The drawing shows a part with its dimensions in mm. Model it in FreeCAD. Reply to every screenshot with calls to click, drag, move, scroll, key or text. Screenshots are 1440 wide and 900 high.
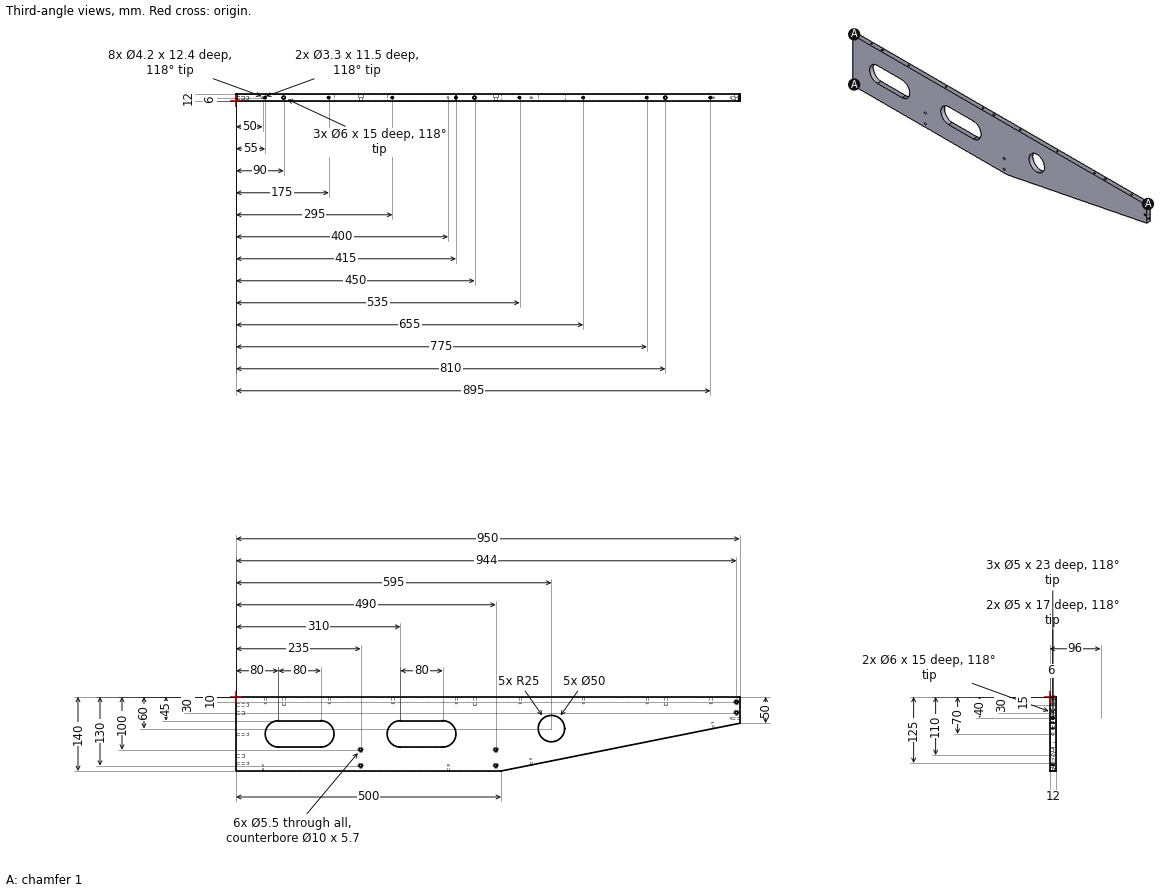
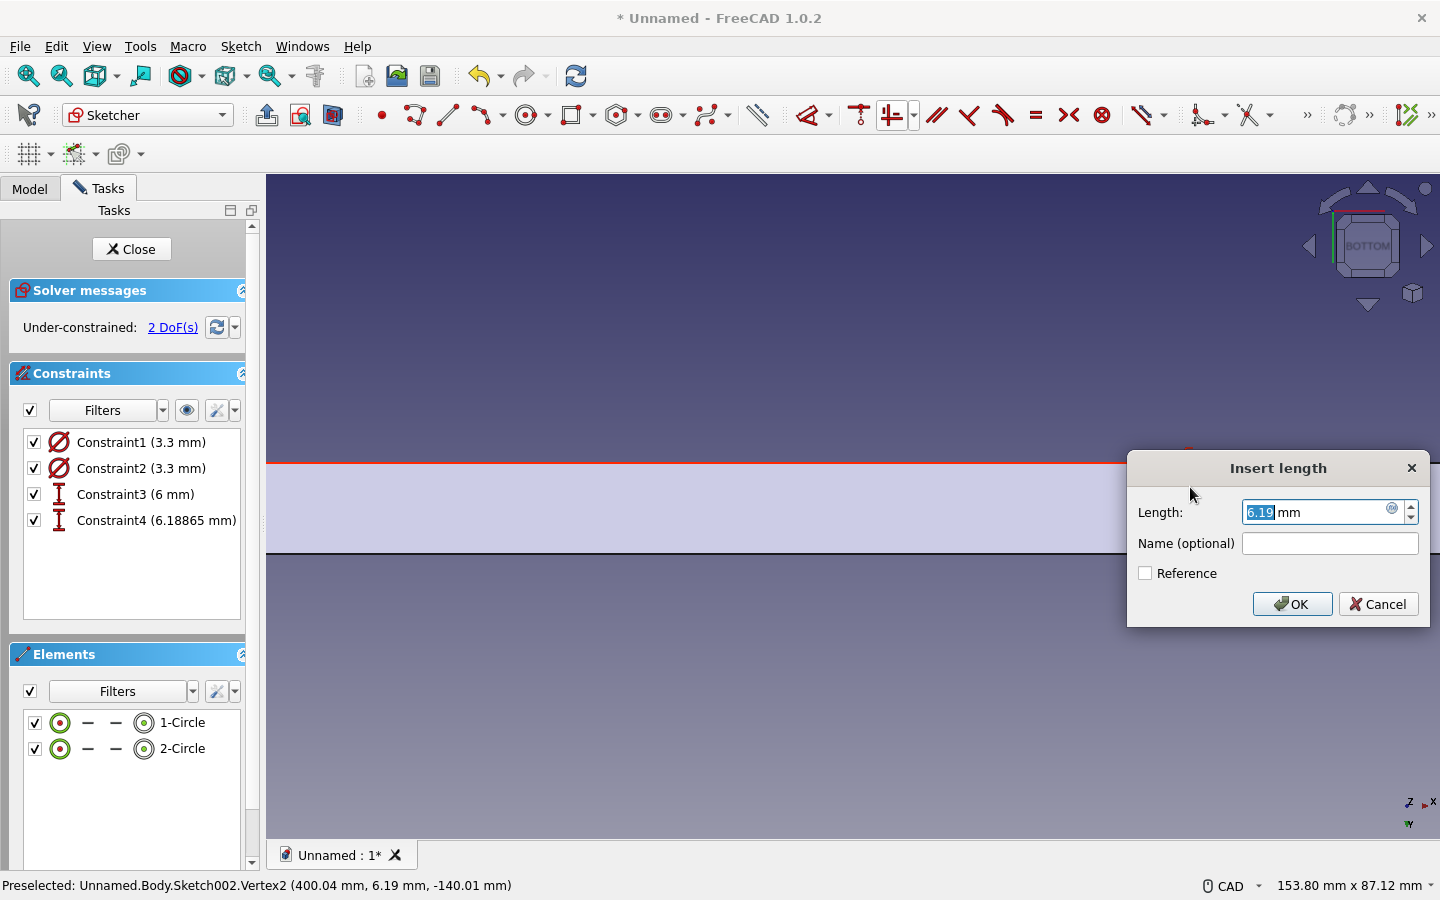
text(6)
key(Return)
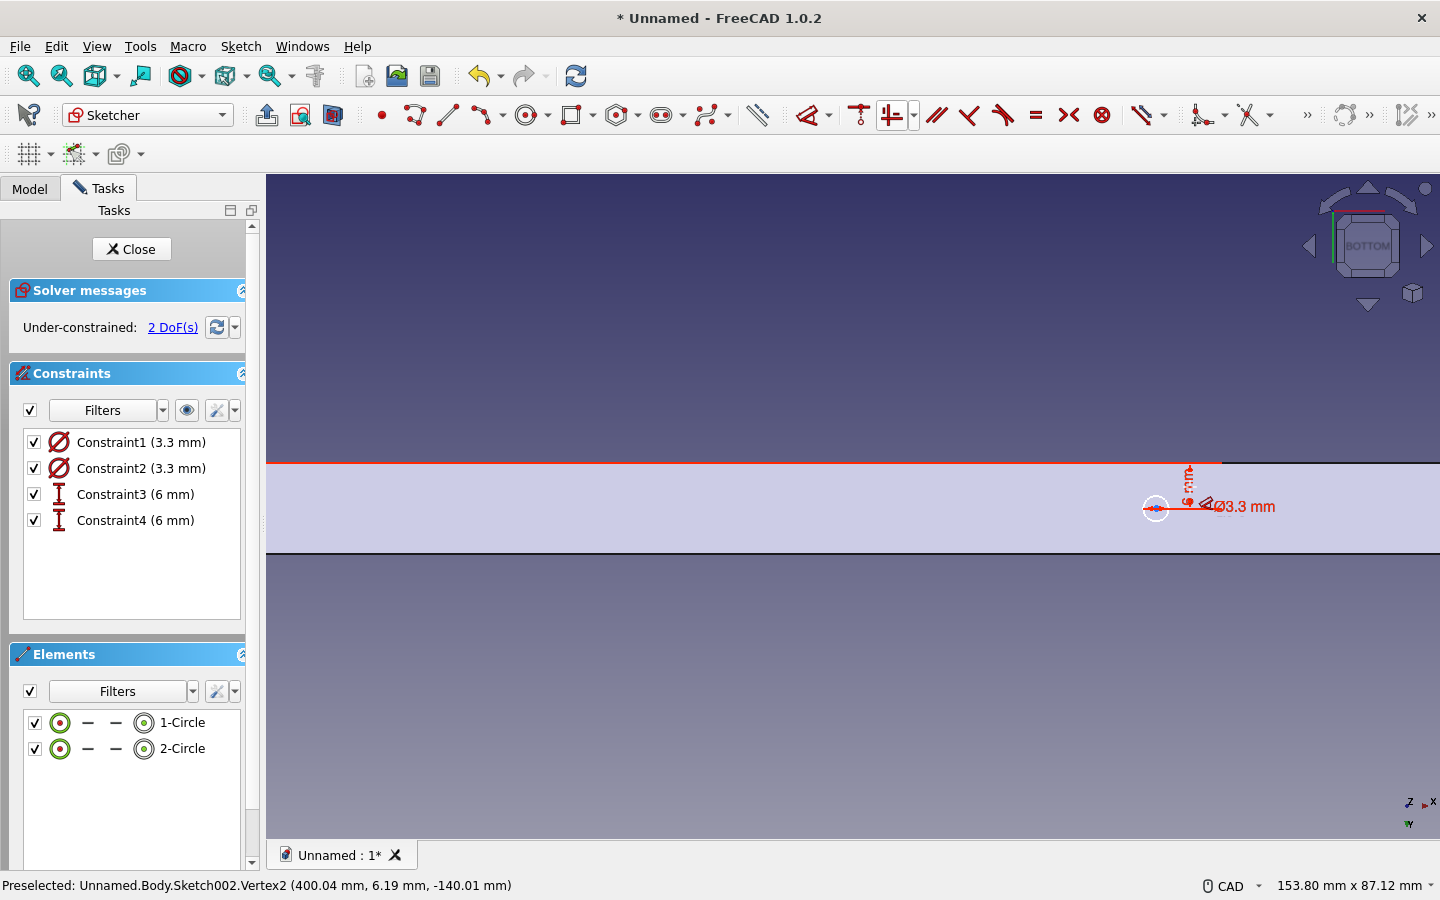
scroll(1161, 511, down, 7)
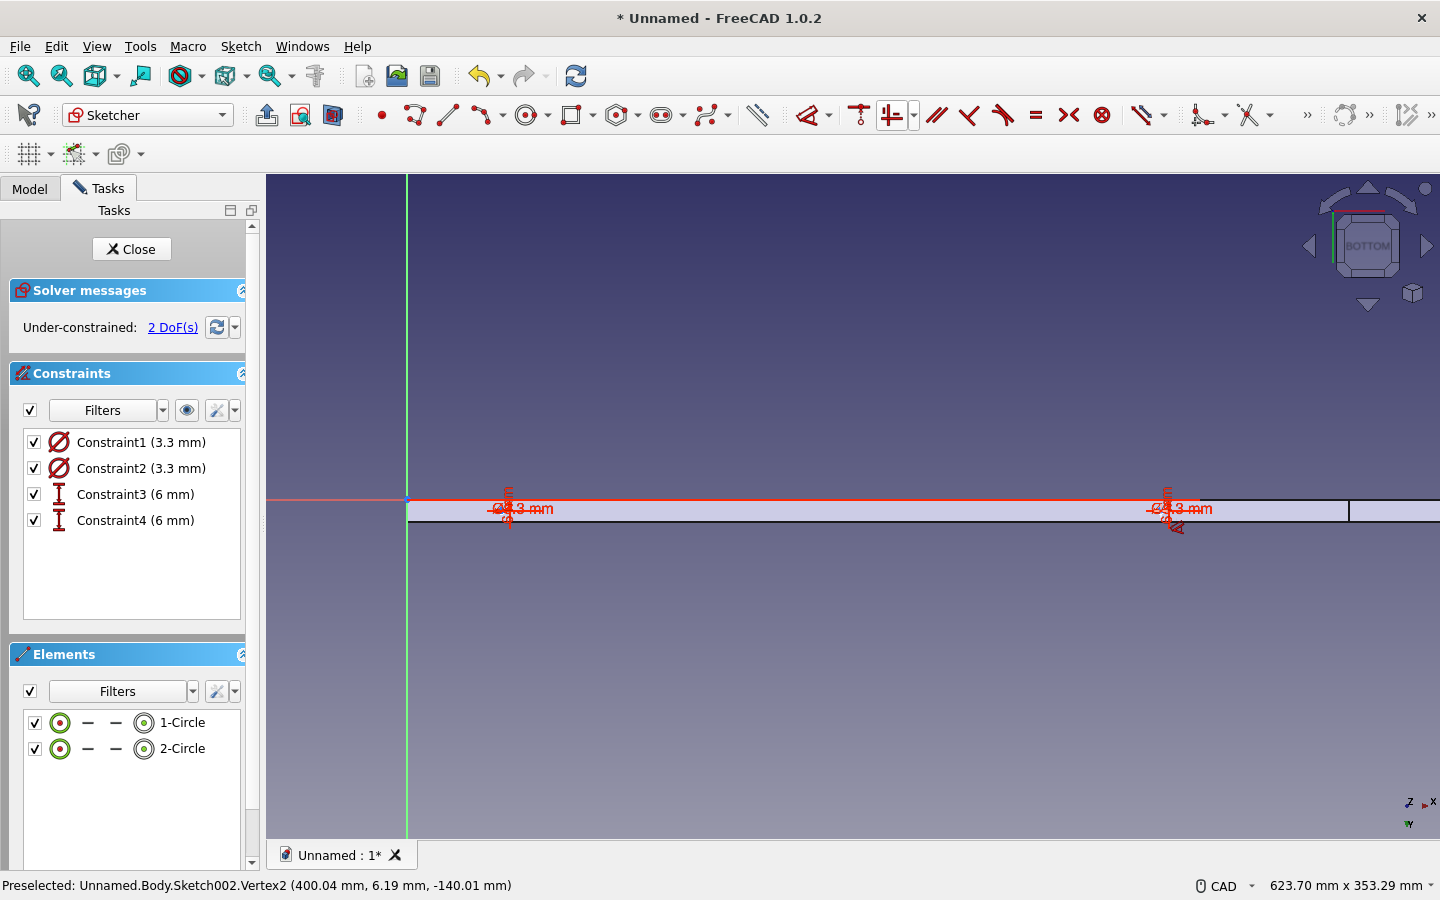
click(501, 511)
click(454, 466)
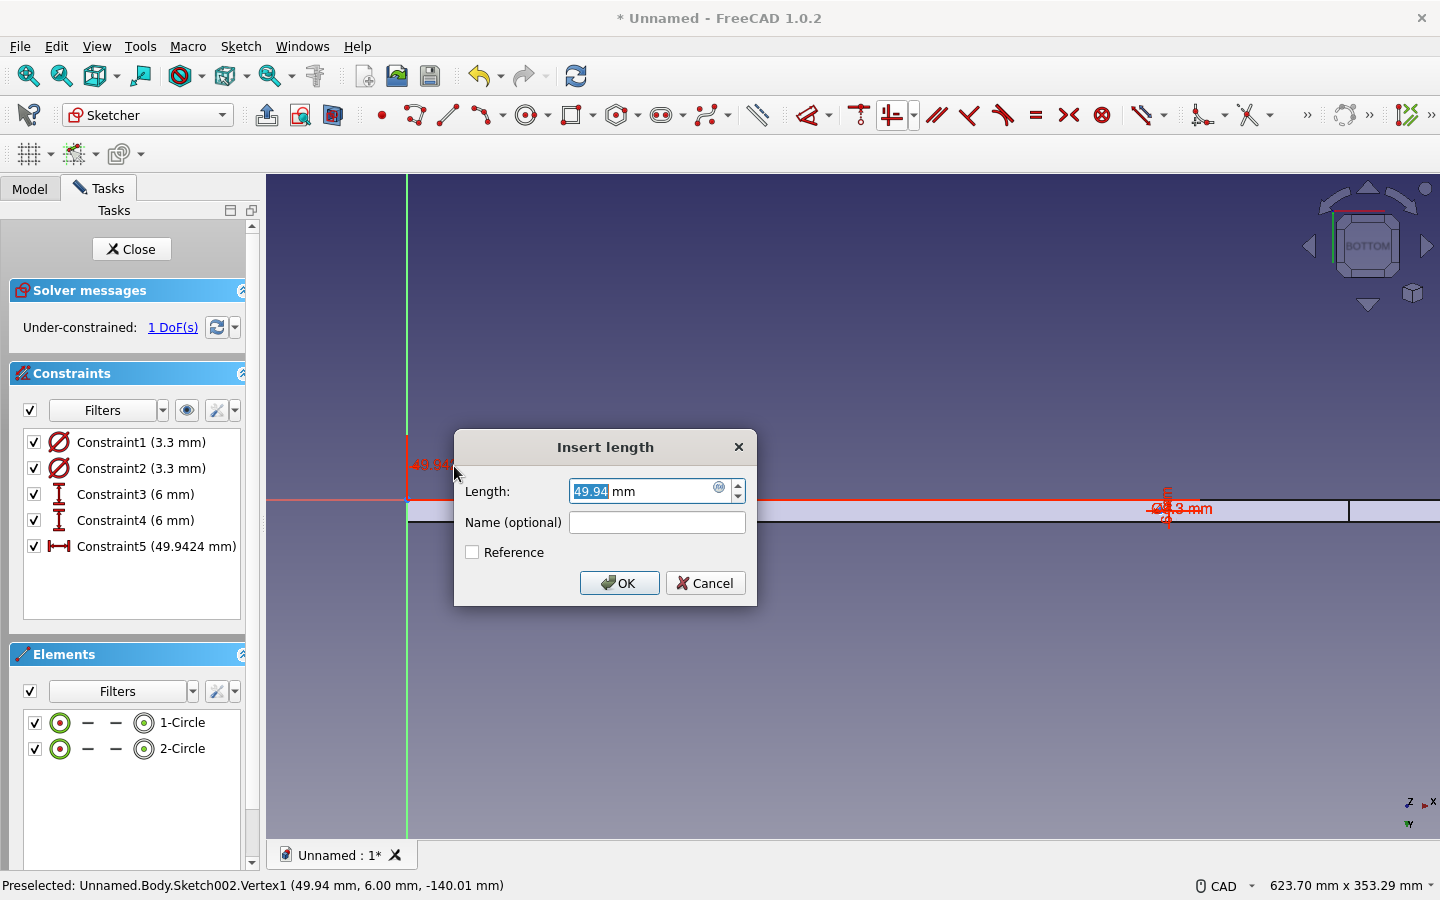
text(50)
key(Return)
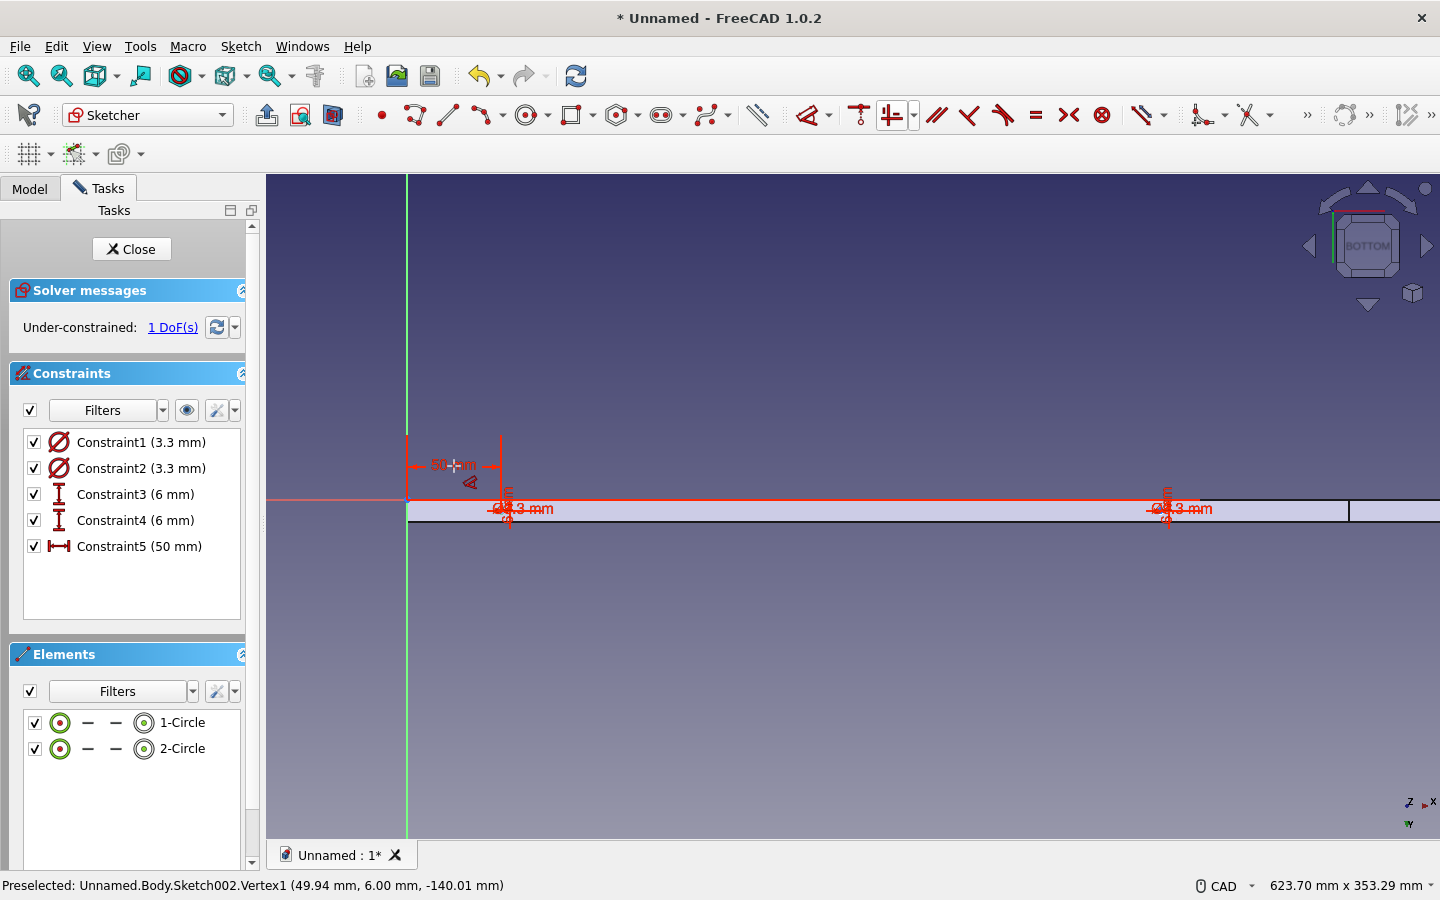
click(1160, 511)
click(784, 466)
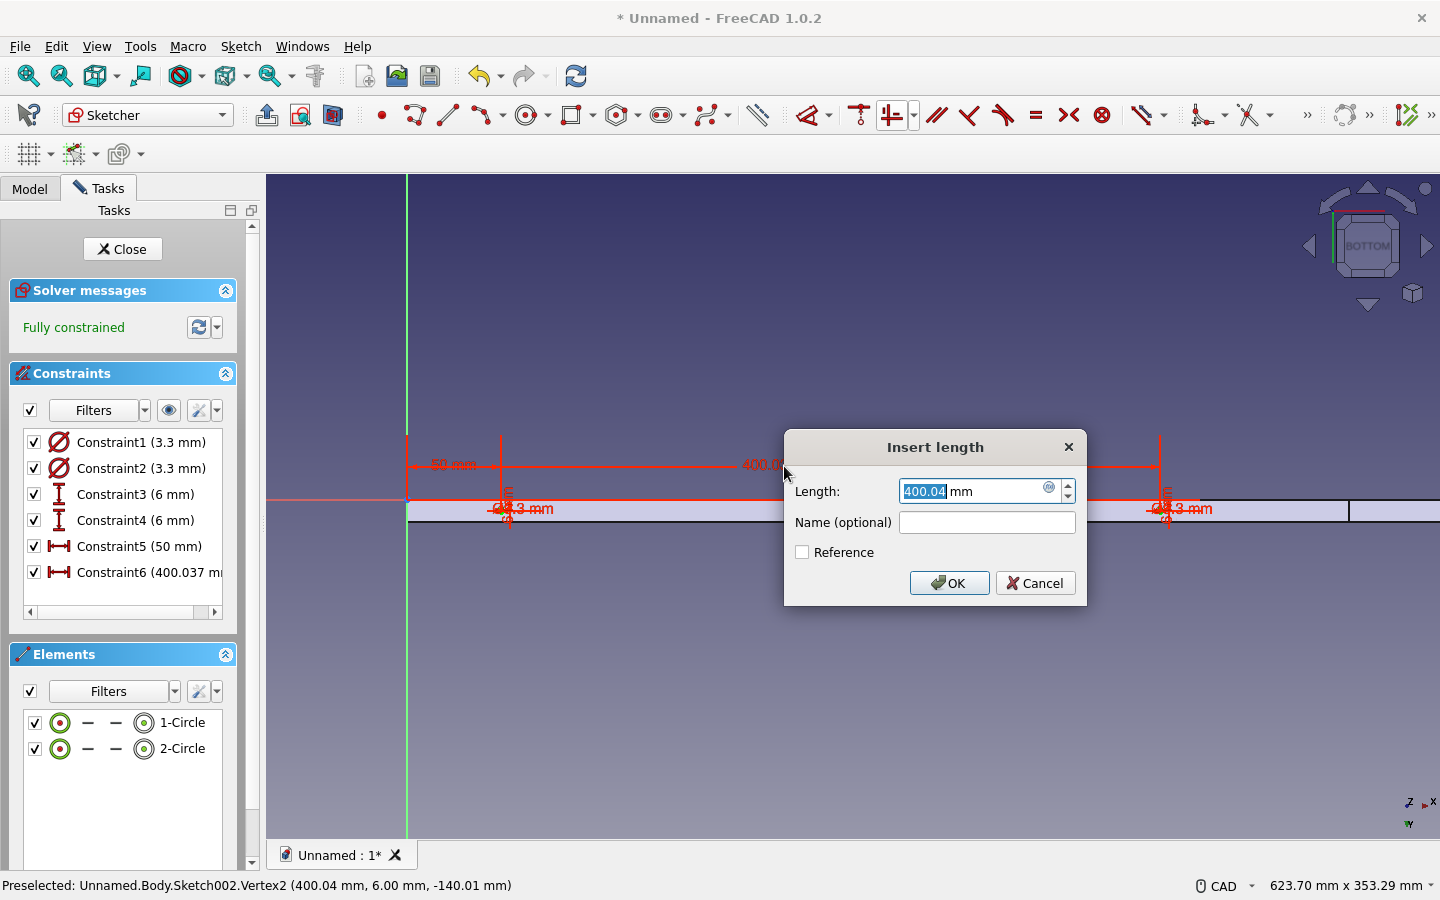
text(400)
key(Return)
key(Escape)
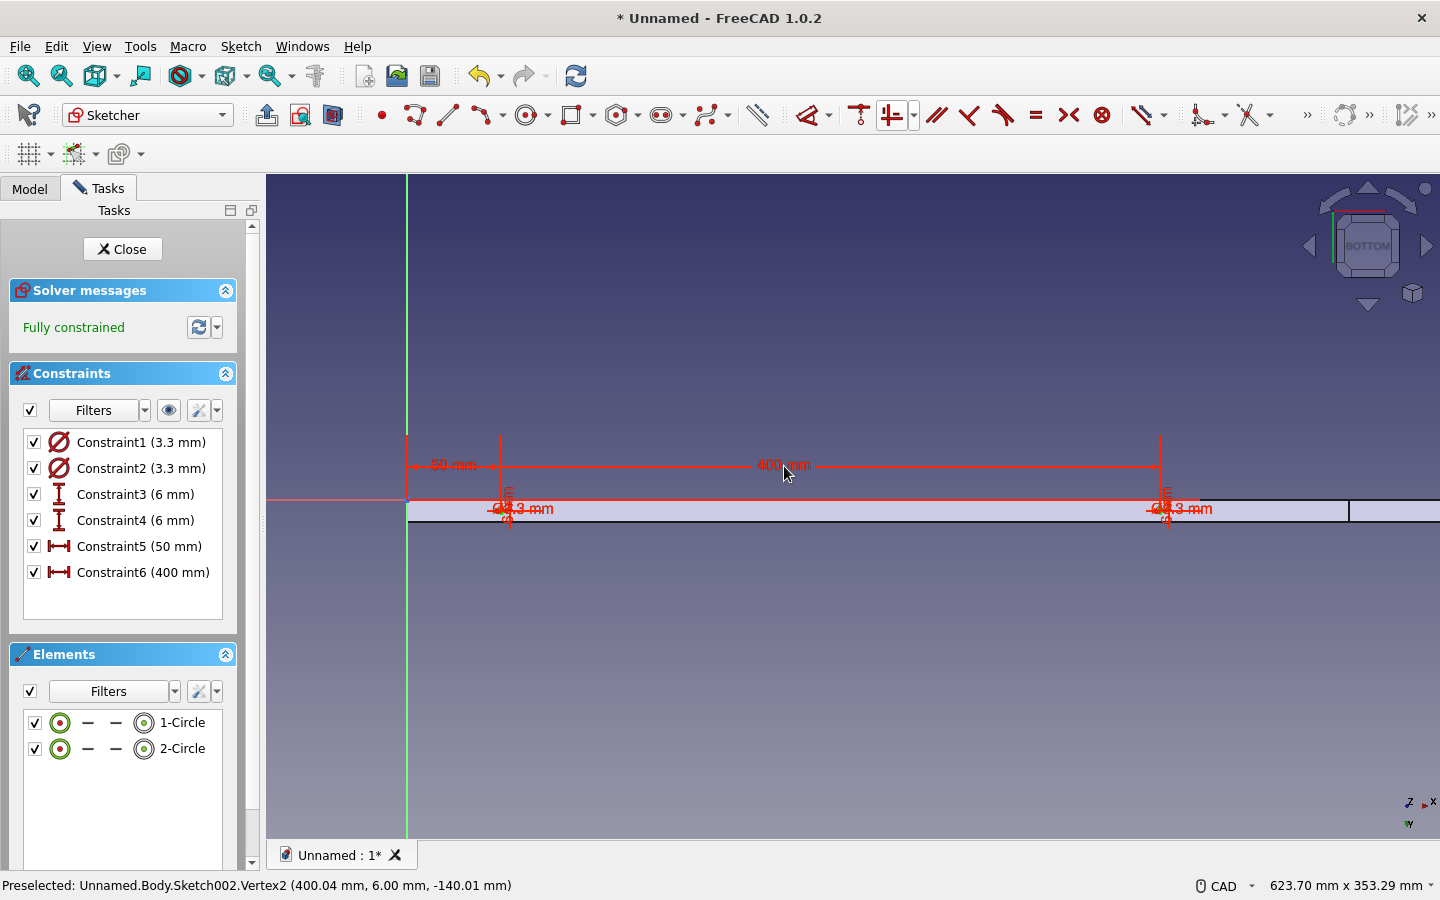
click(123, 249)